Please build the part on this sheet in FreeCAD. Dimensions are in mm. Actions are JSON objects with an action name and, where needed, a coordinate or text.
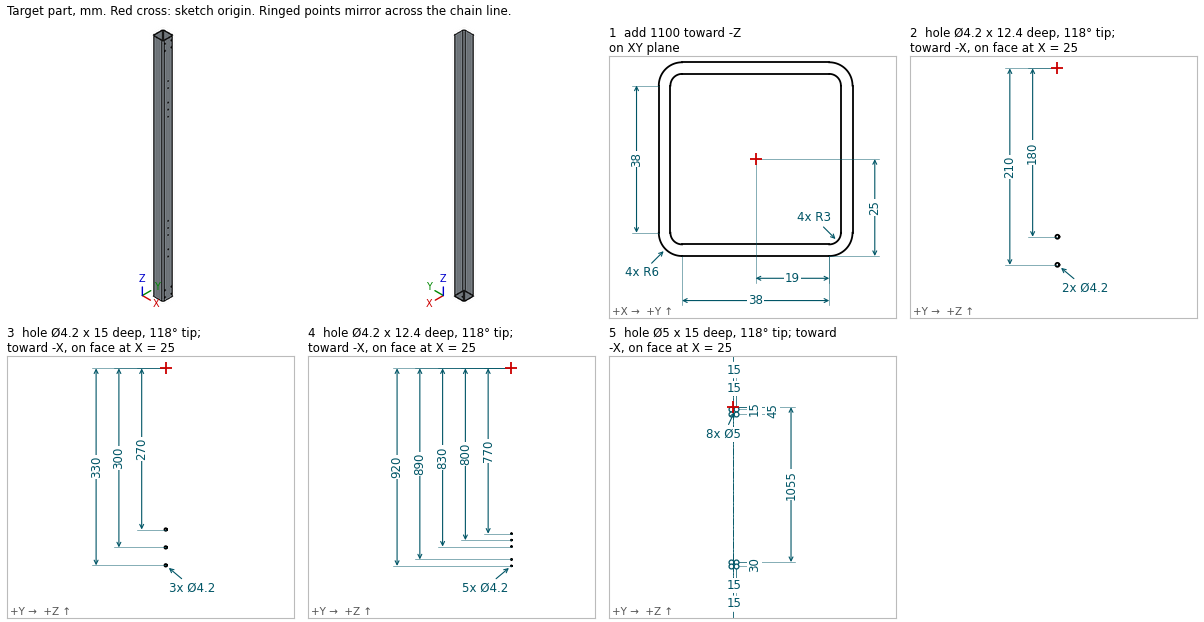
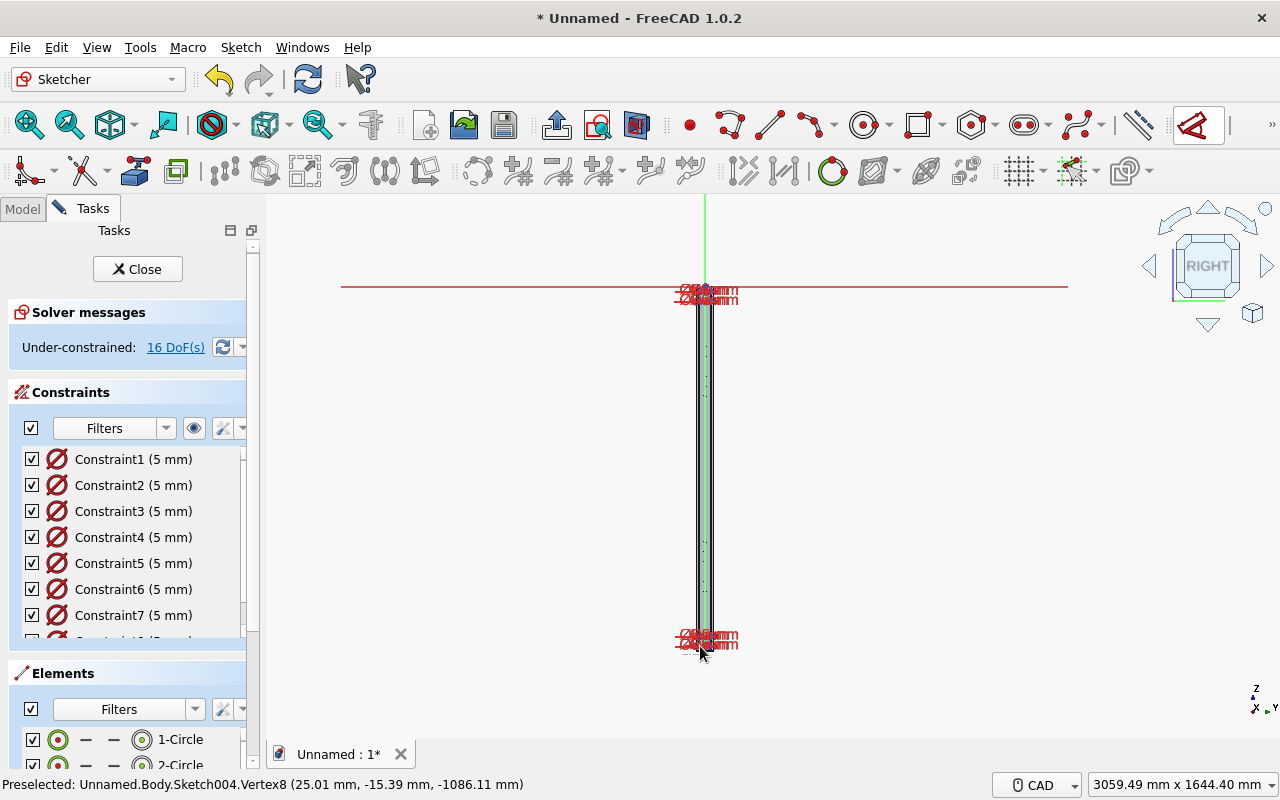
{"action": "scroll", "coordinate": [710, 292], "scroll_direction": "up", "scroll_amount": 3}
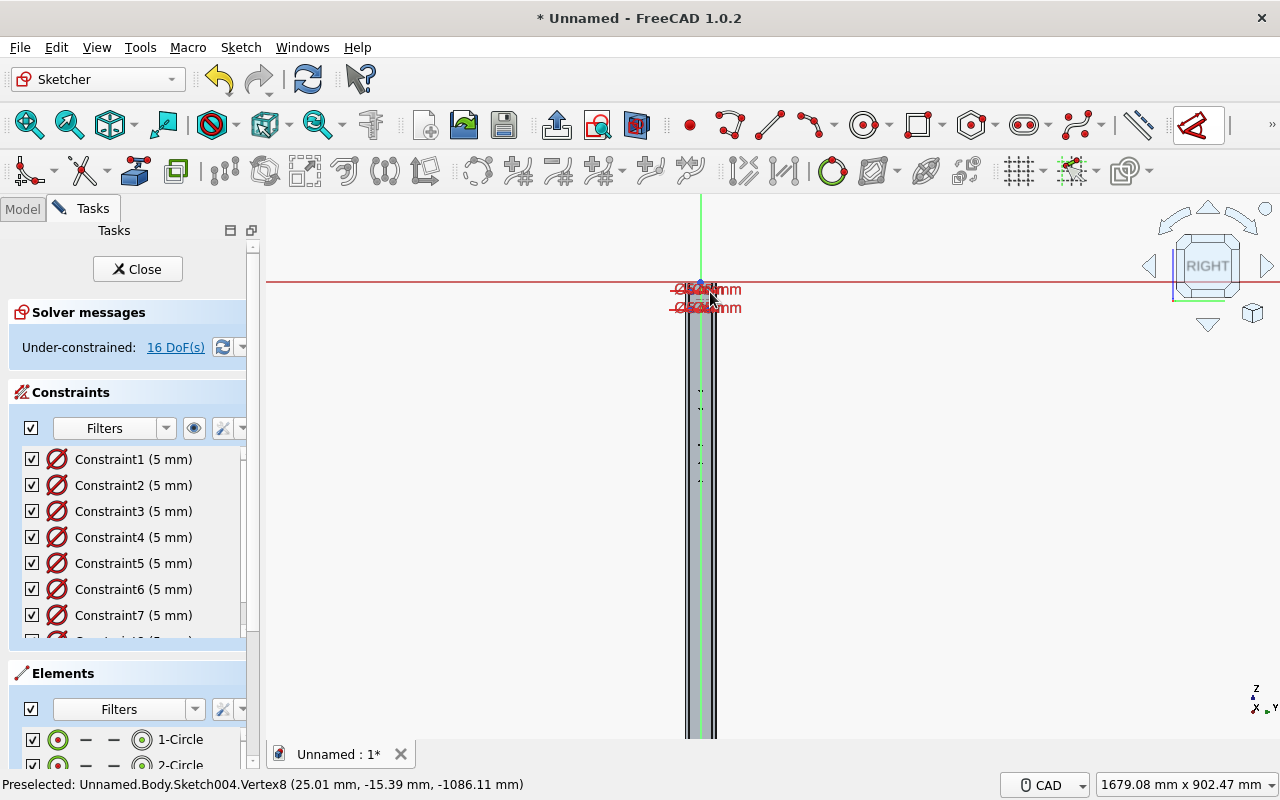
{"action": "left_click", "coordinate": [710, 292]}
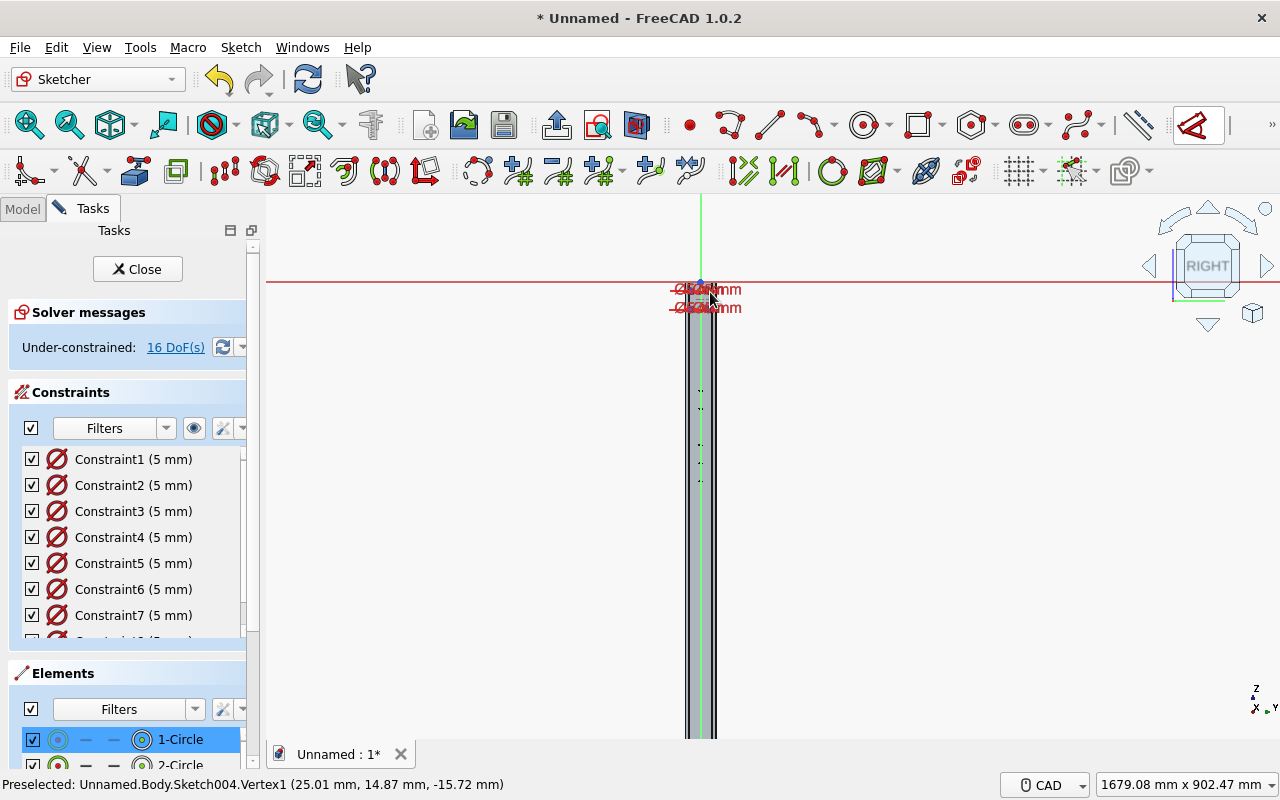
{"action": "left_click", "coordinate": [691, 291]}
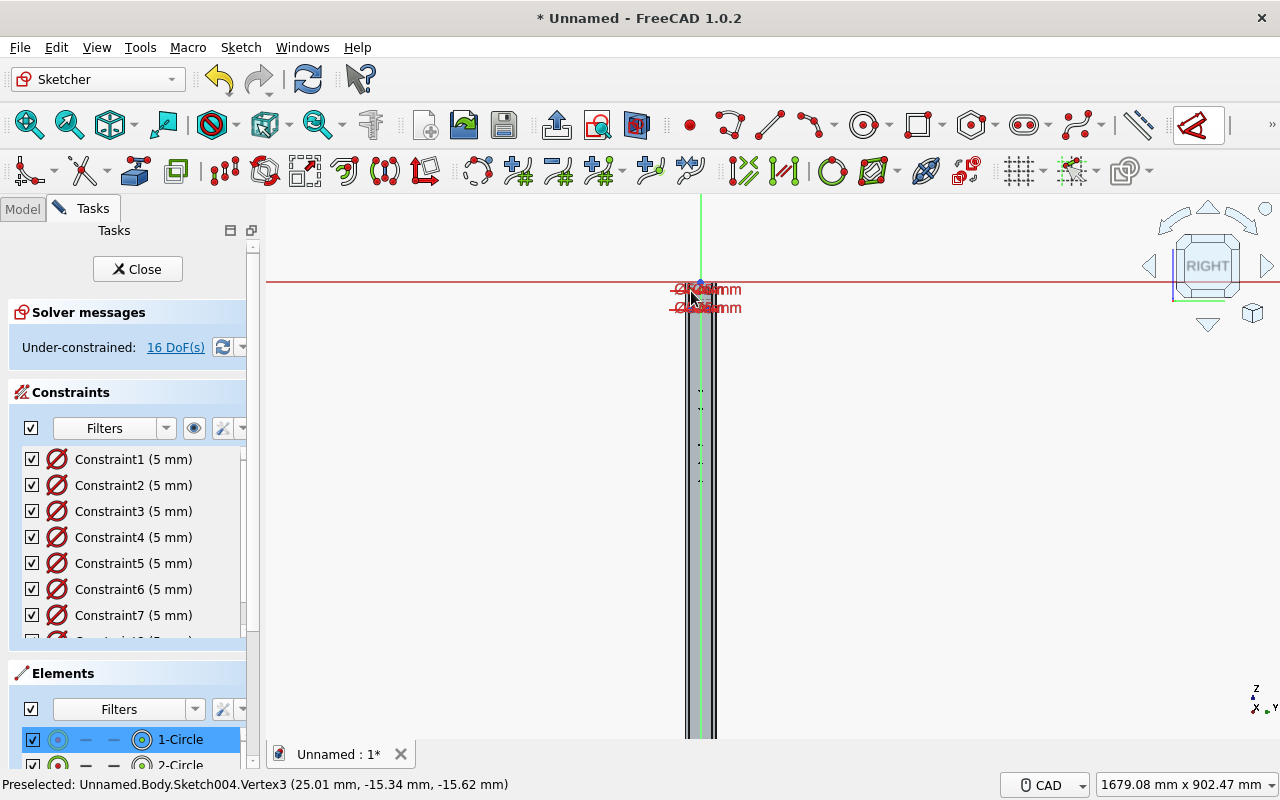
{"action": "left_click", "coordinate": [701, 676]}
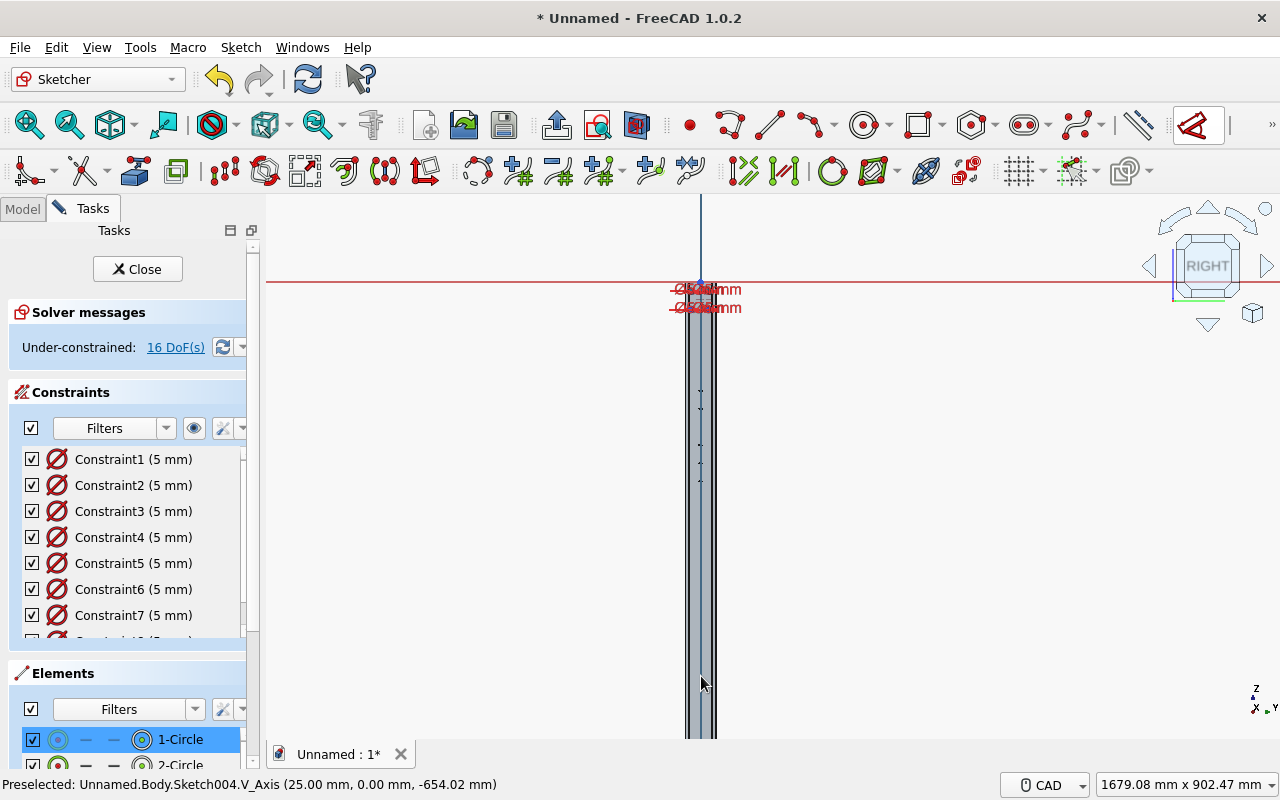
{"action": "key", "text": "s"}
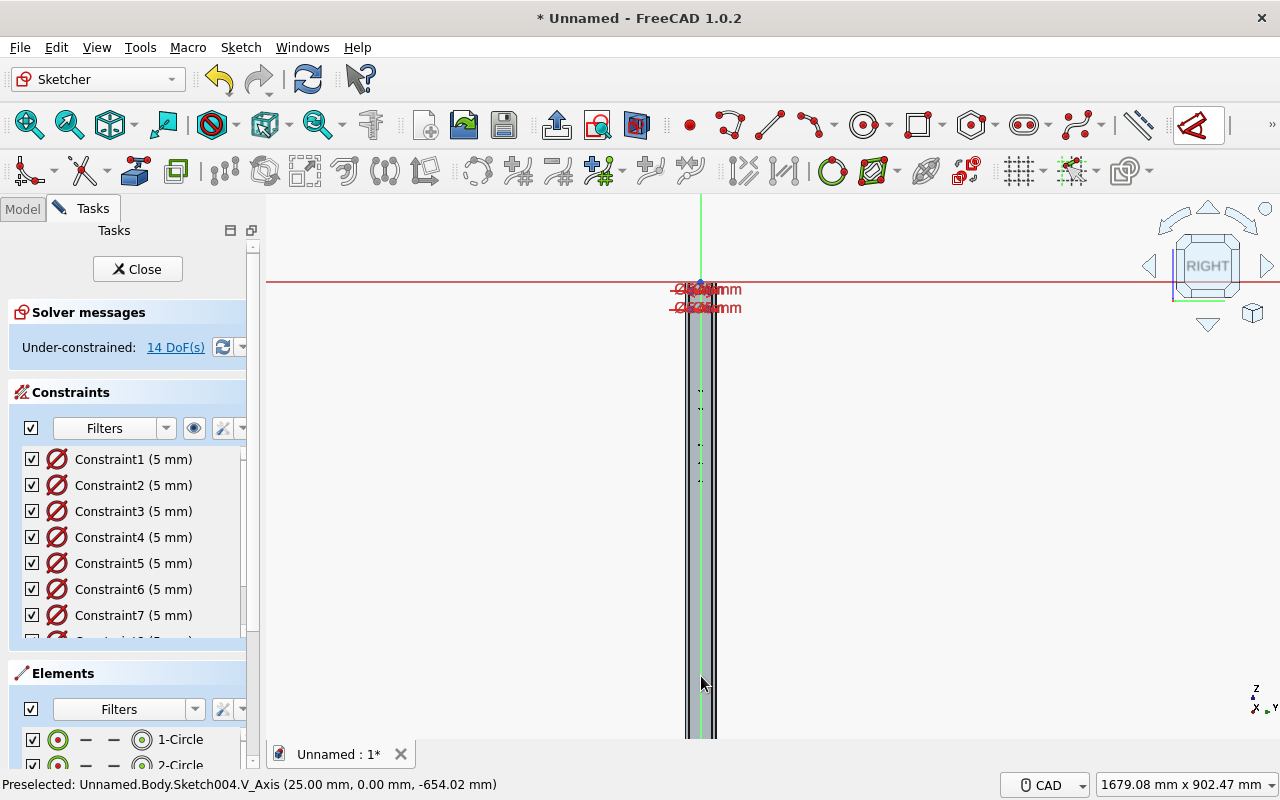
{"action": "left_click", "coordinate": [710, 310]}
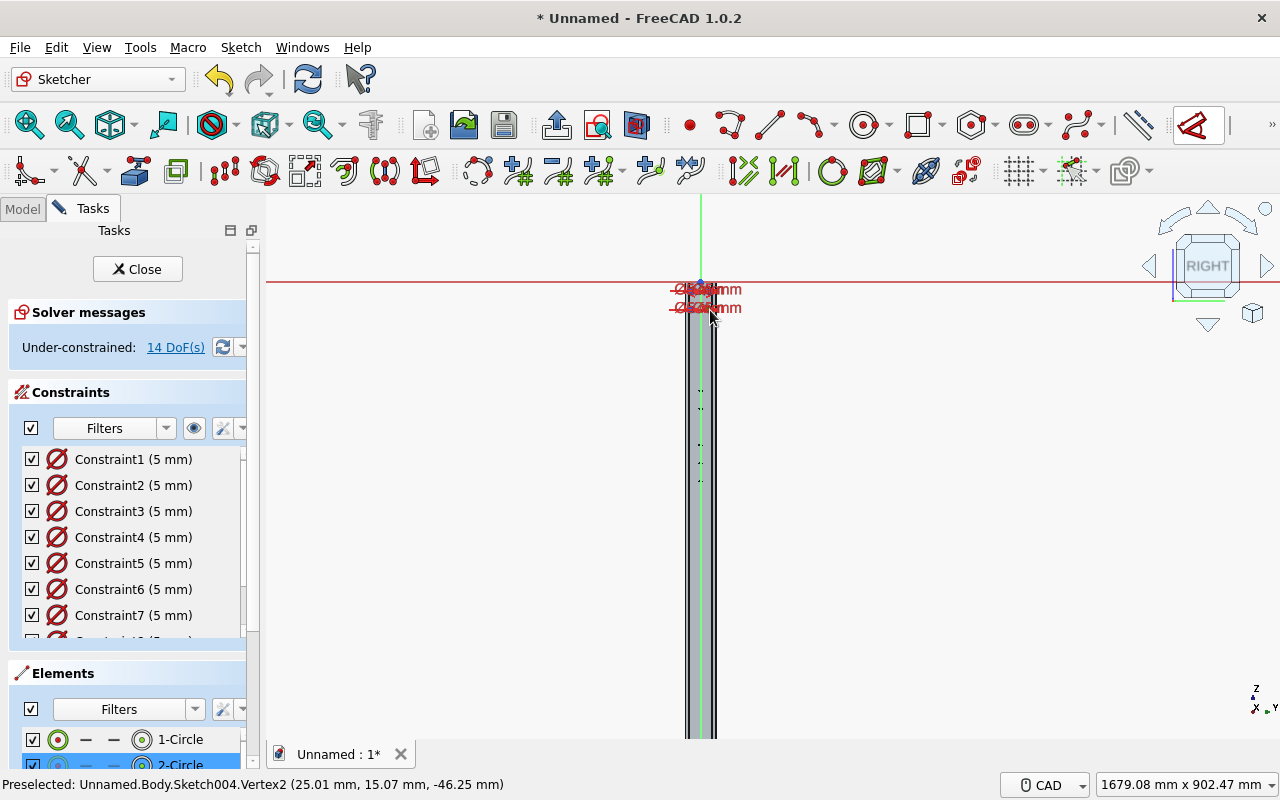
{"action": "left_click", "coordinate": [692, 310]}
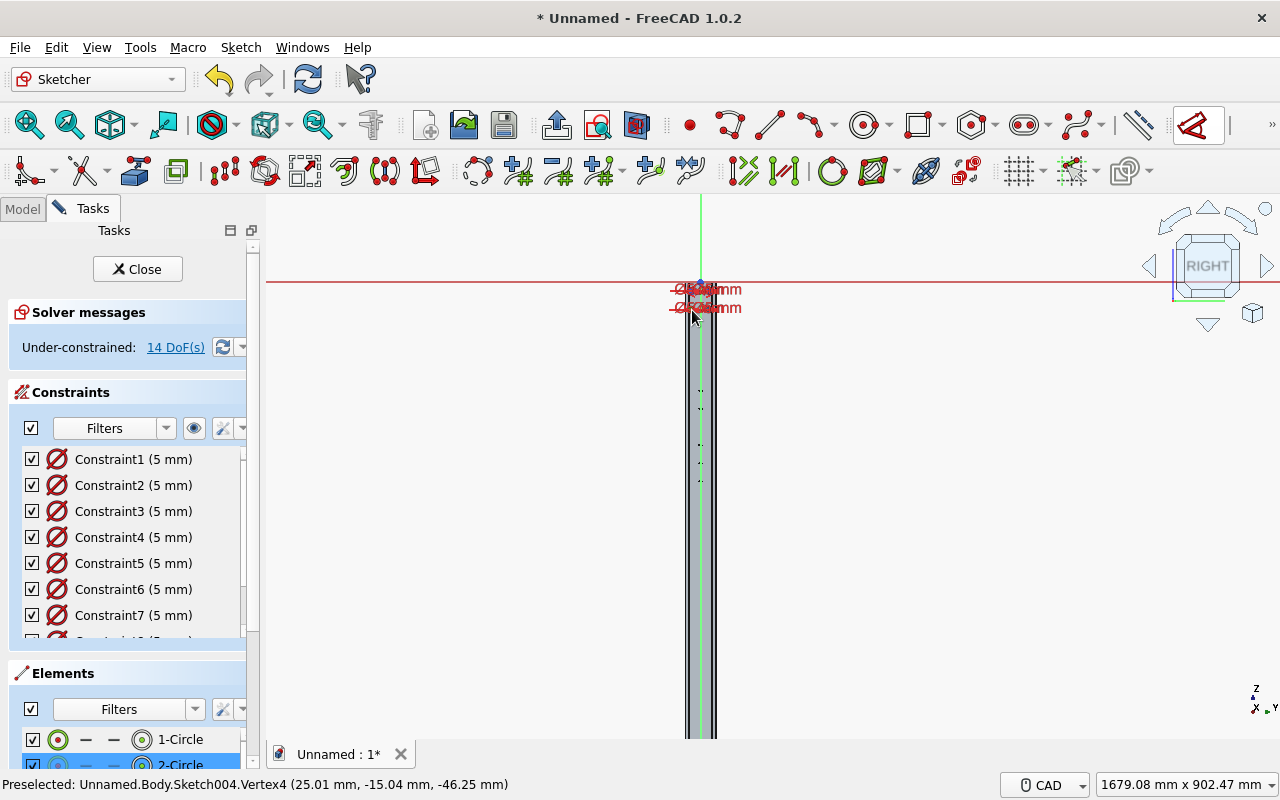
{"action": "left_click", "coordinate": [701, 676]}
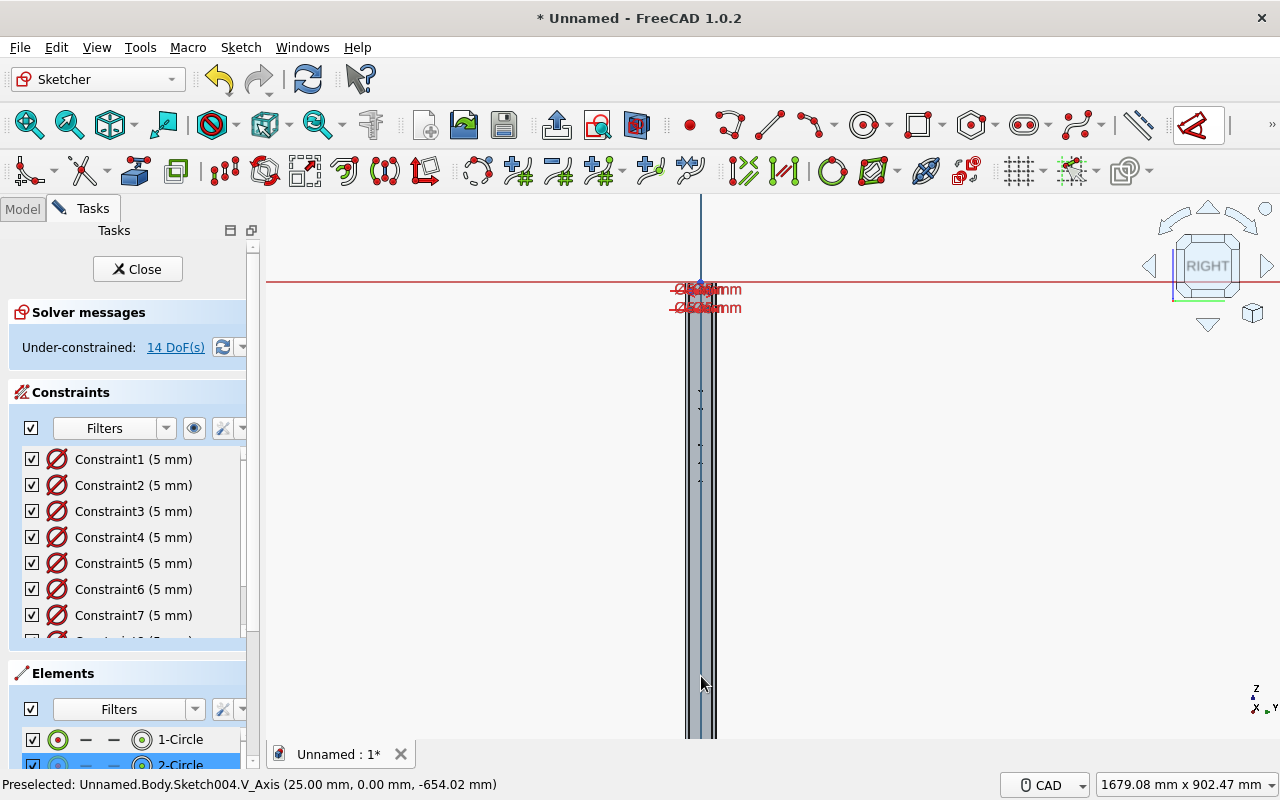
{"action": "key", "text": "s"}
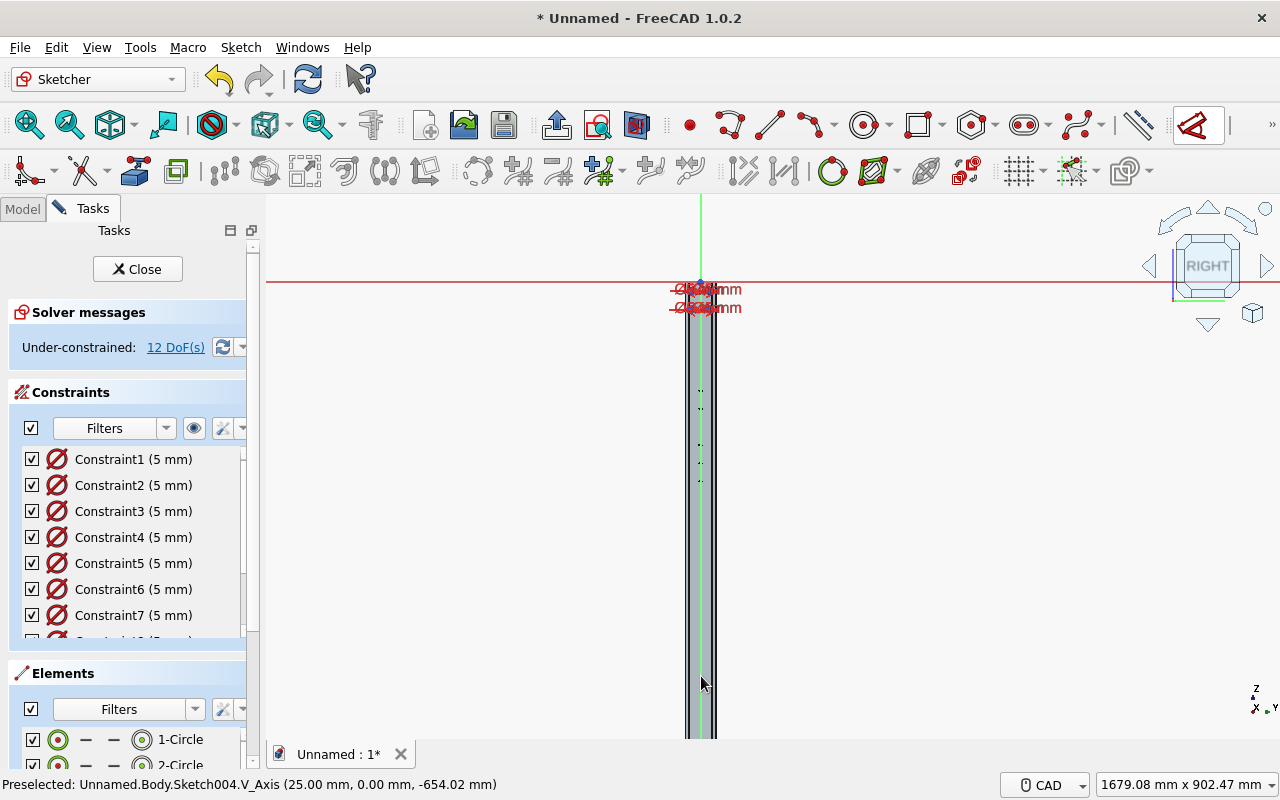
{"action": "scroll", "coordinate": [709, 291], "scroll_direction": "down", "scroll_amount": 3}